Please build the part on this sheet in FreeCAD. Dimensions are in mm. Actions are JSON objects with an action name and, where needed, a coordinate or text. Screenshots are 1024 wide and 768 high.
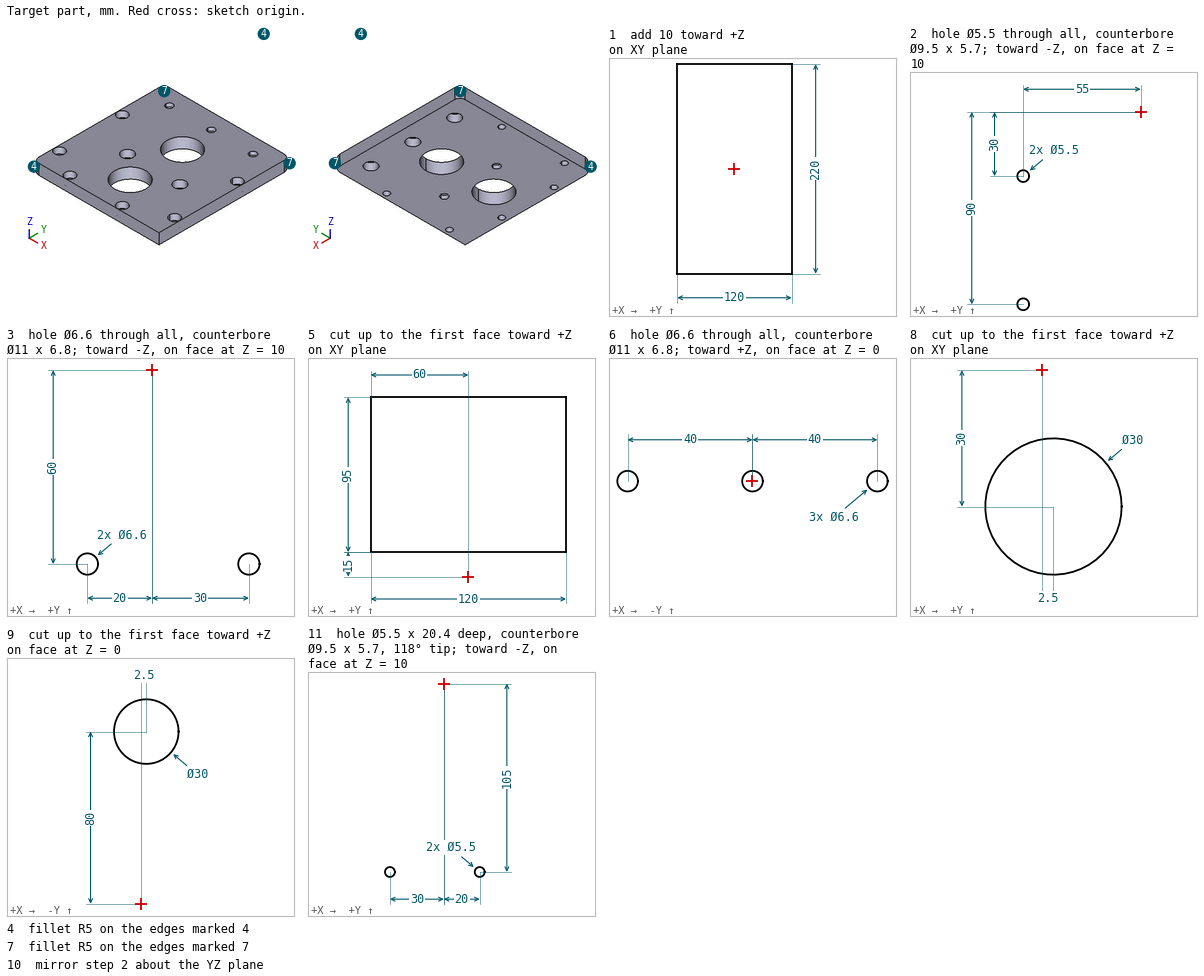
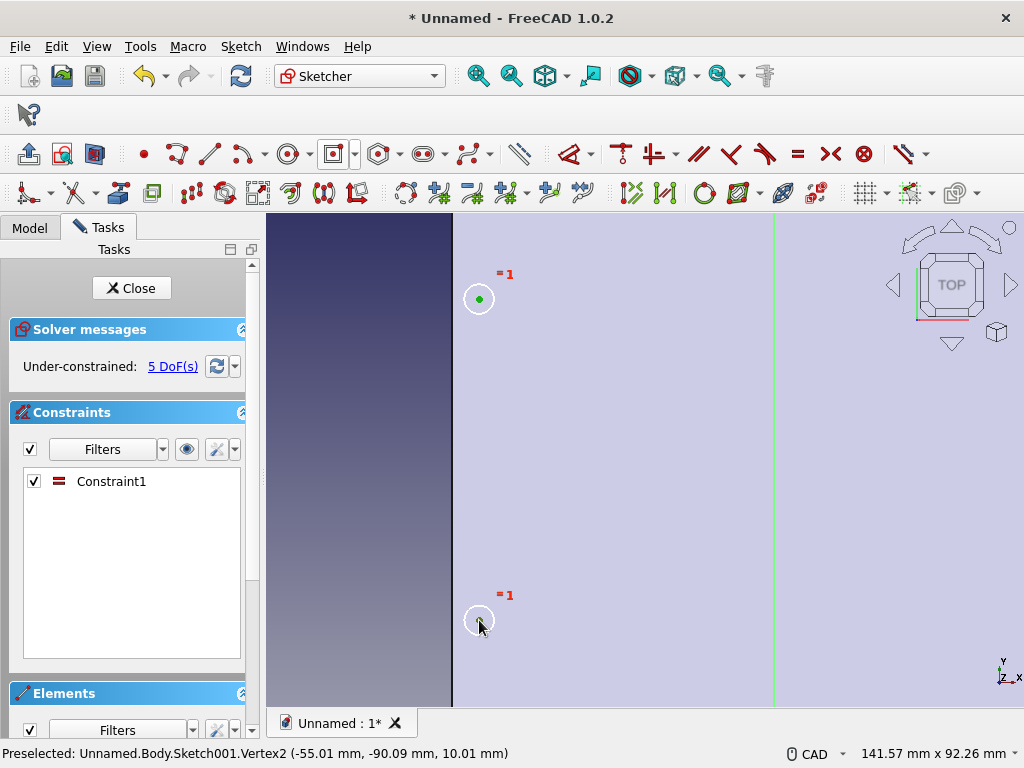
{"action": "key", "text": "v"}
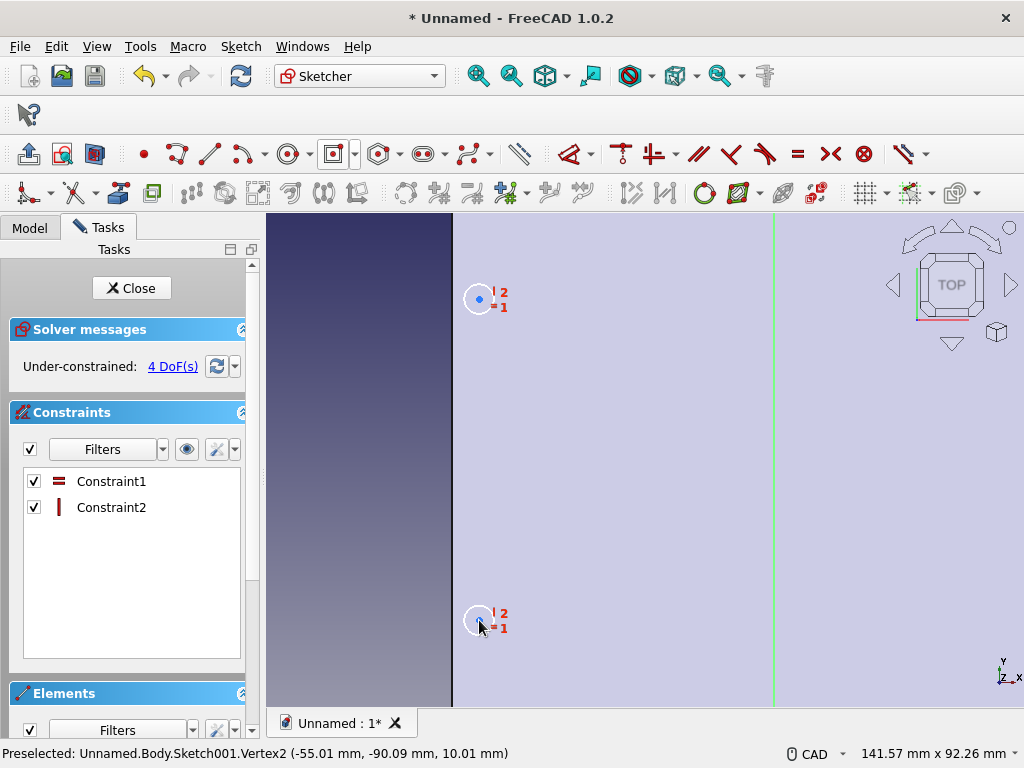
{"action": "left_click", "coordinate": [568, 154]}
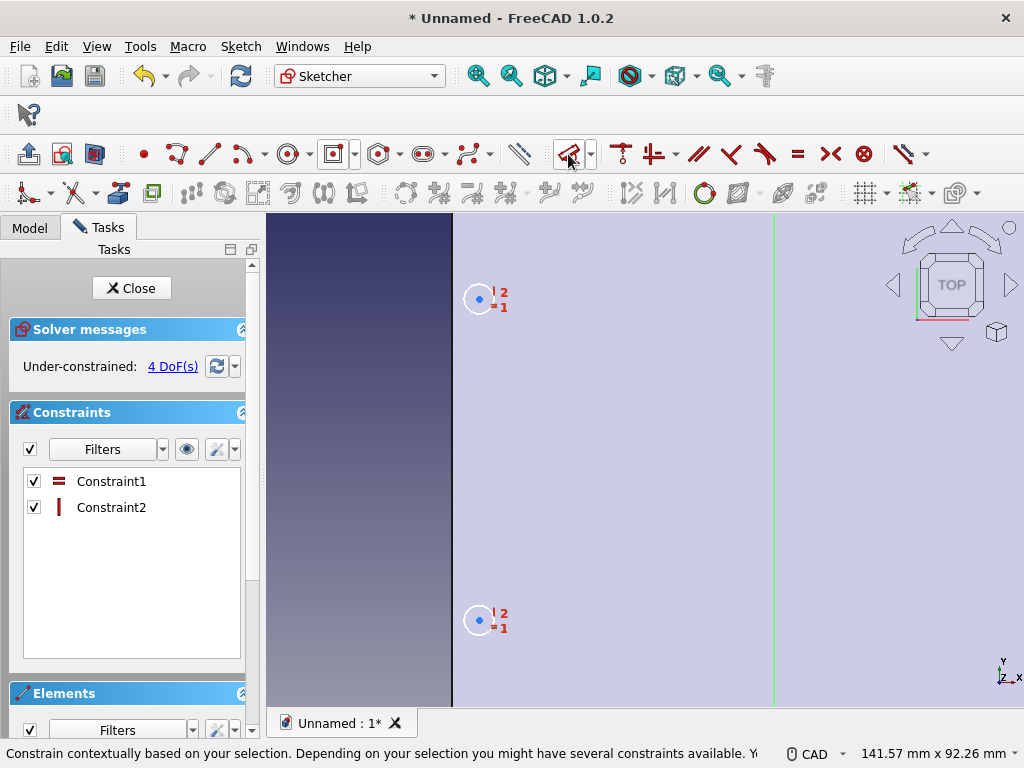
{"action": "scroll", "coordinate": [489, 289], "scroll_direction": "up", "scroll_amount": 2}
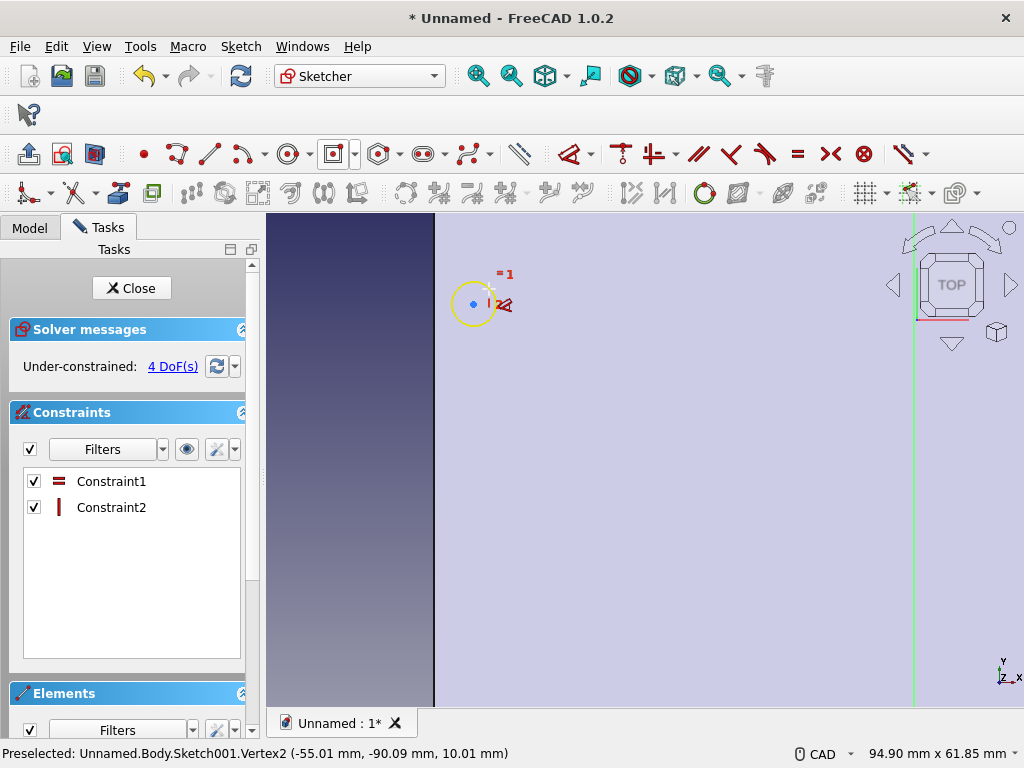
{"action": "left_click", "coordinate": [489, 288]}
{"action": "left_click", "coordinate": [511, 265]}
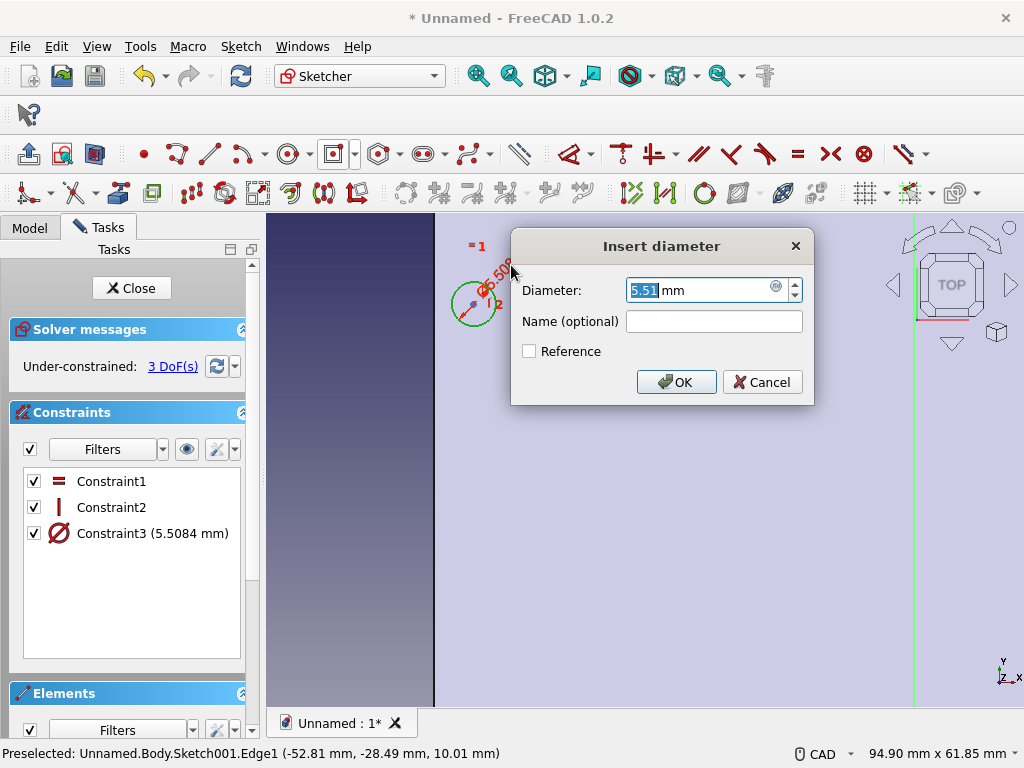
{"action": "type", "text": "5.5"}
{"action": "key", "text": "Return"}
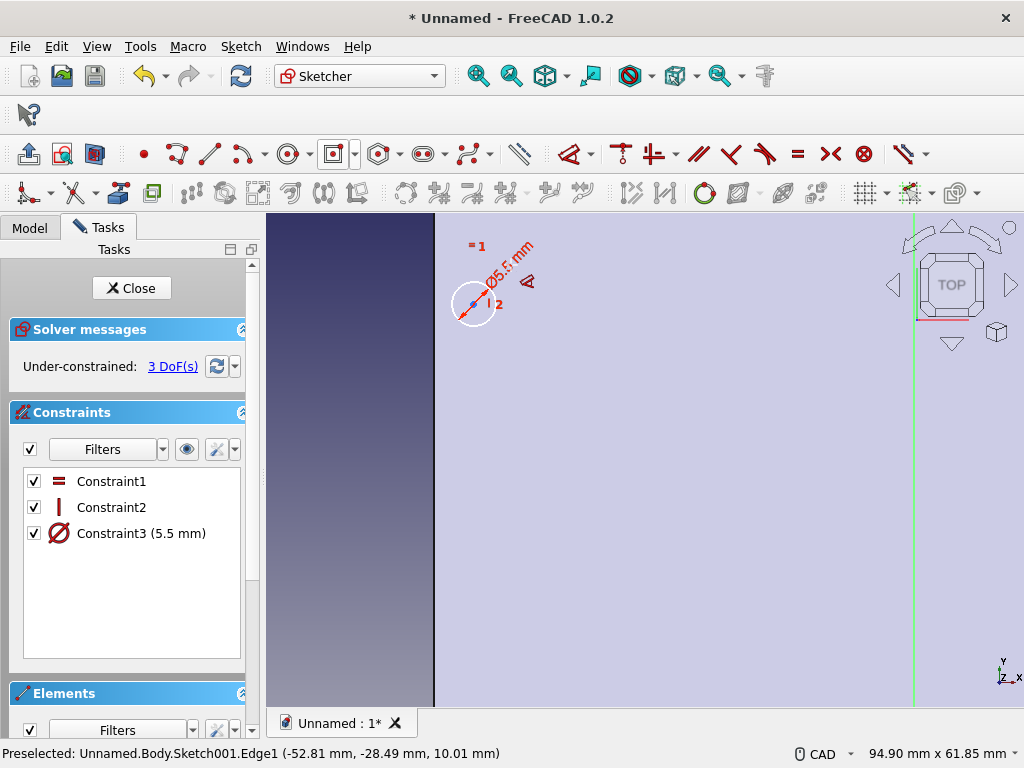
{"action": "left_click", "coordinate": [474, 304]}
{"action": "left_click", "coordinate": [666, 338]}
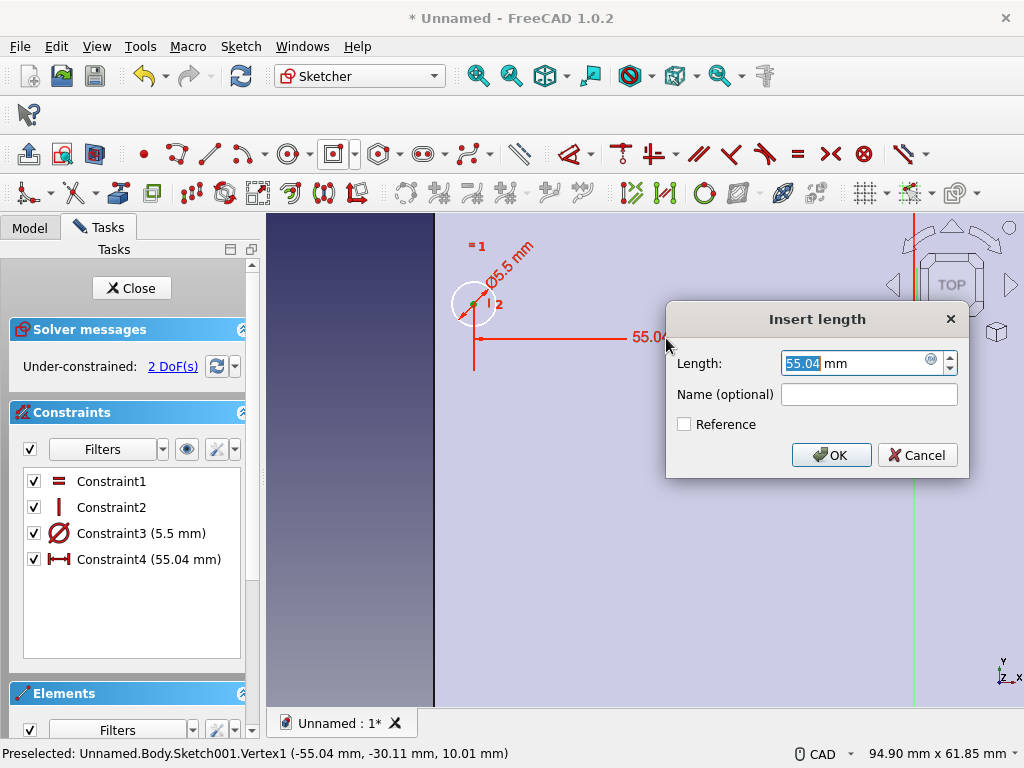
{"action": "type", "text": "55"}
{"action": "key", "text": "Return"}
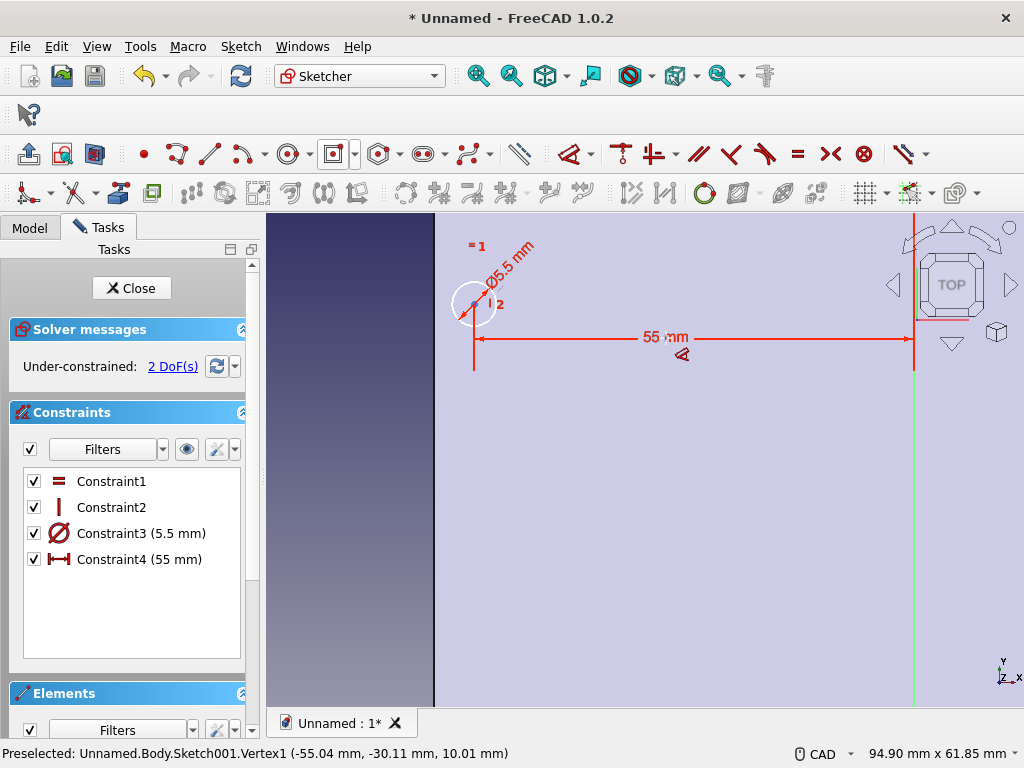
{"action": "left_click", "coordinate": [474, 304]}
{"action": "left_click", "coordinate": [440, 273]}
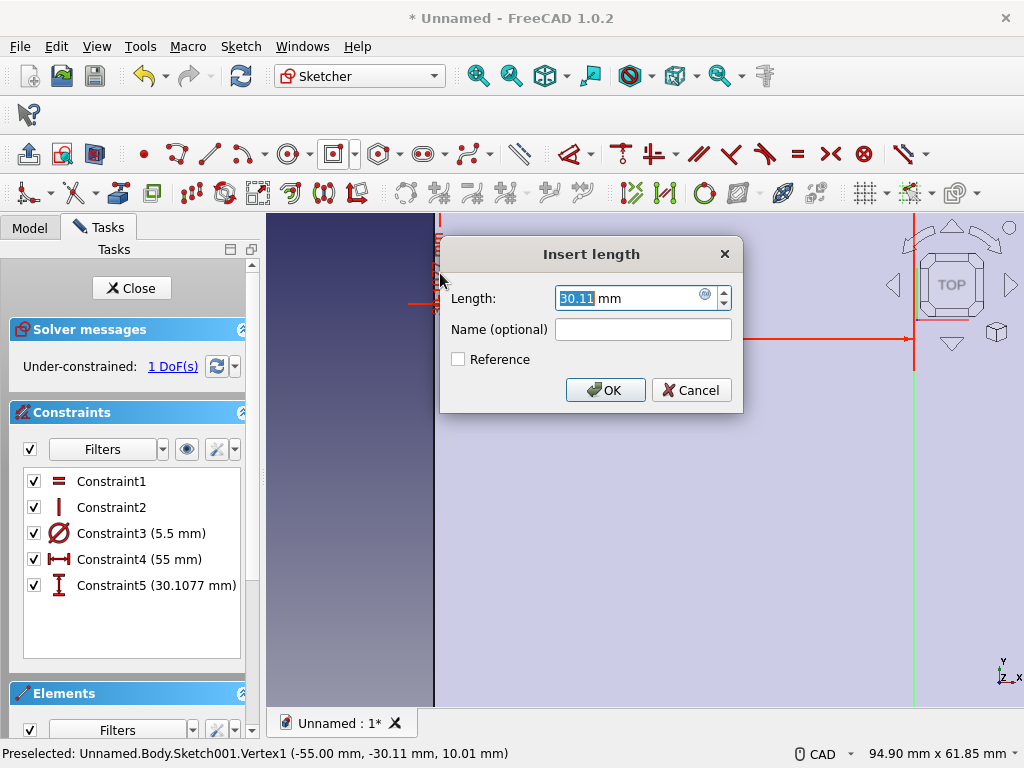
{"action": "type", "text": "30"}
{"action": "key", "text": "Return"}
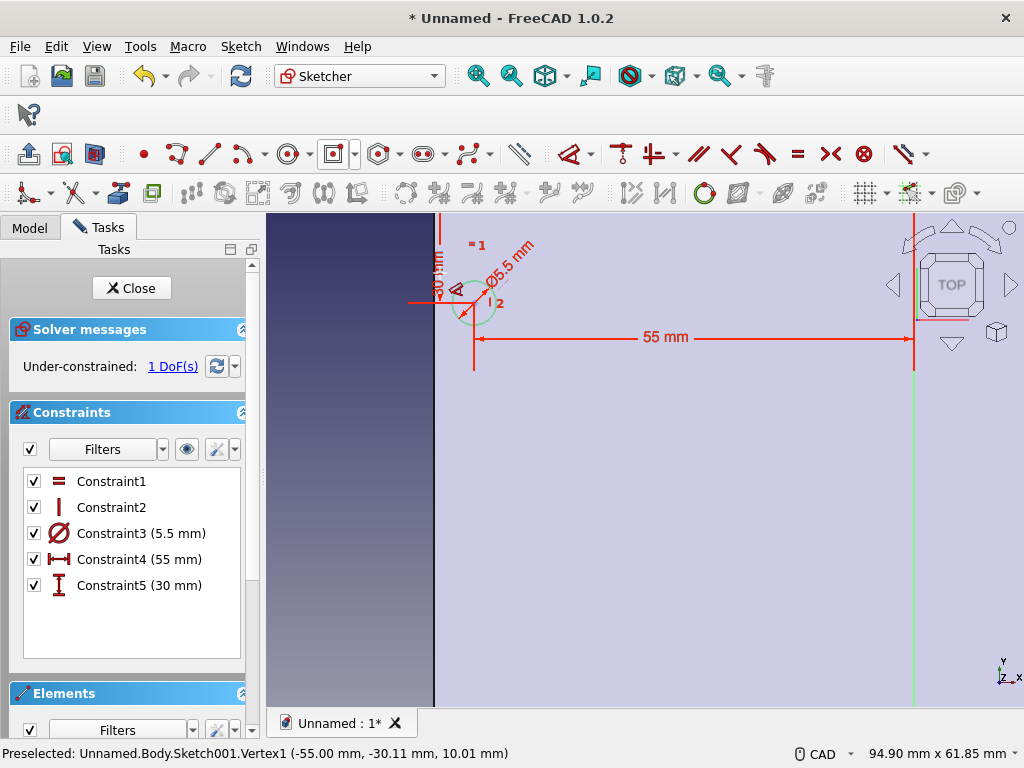
{"action": "scroll", "coordinate": [490, 481], "scroll_direction": "down", "scroll_amount": 4}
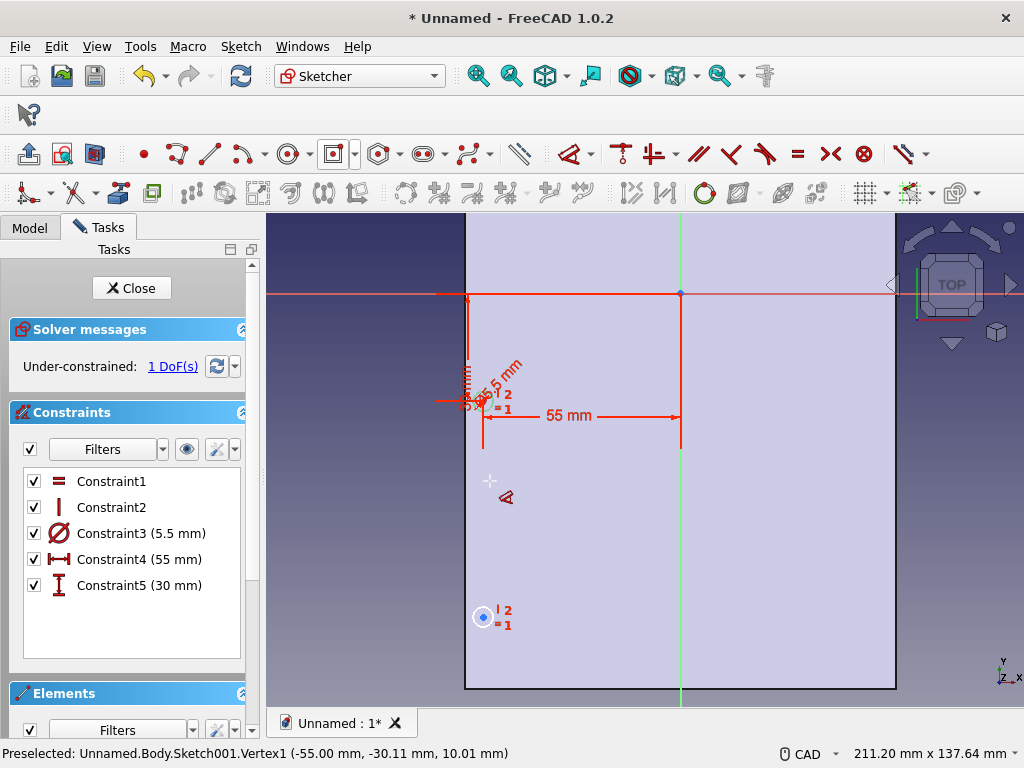
{"action": "left_click", "coordinate": [483, 617]}
{"action": "left_click", "coordinate": [715, 455]}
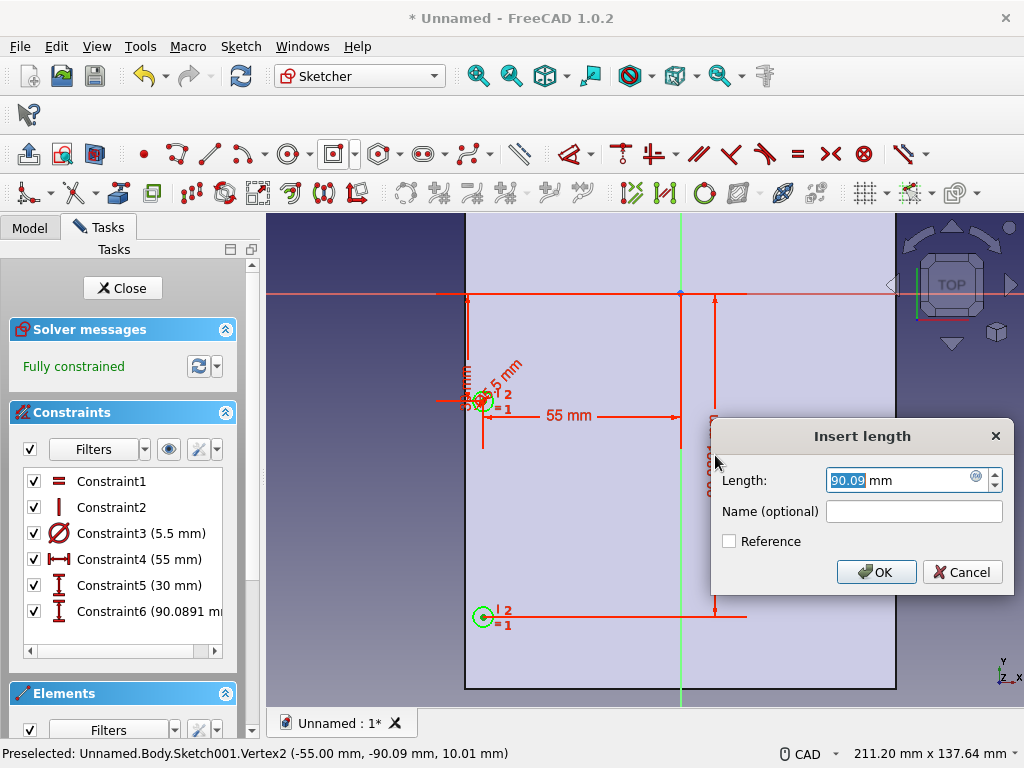
{"action": "type", "text": "90"}
{"action": "key", "text": "Return"}
{"action": "key", "text": "Escape"}